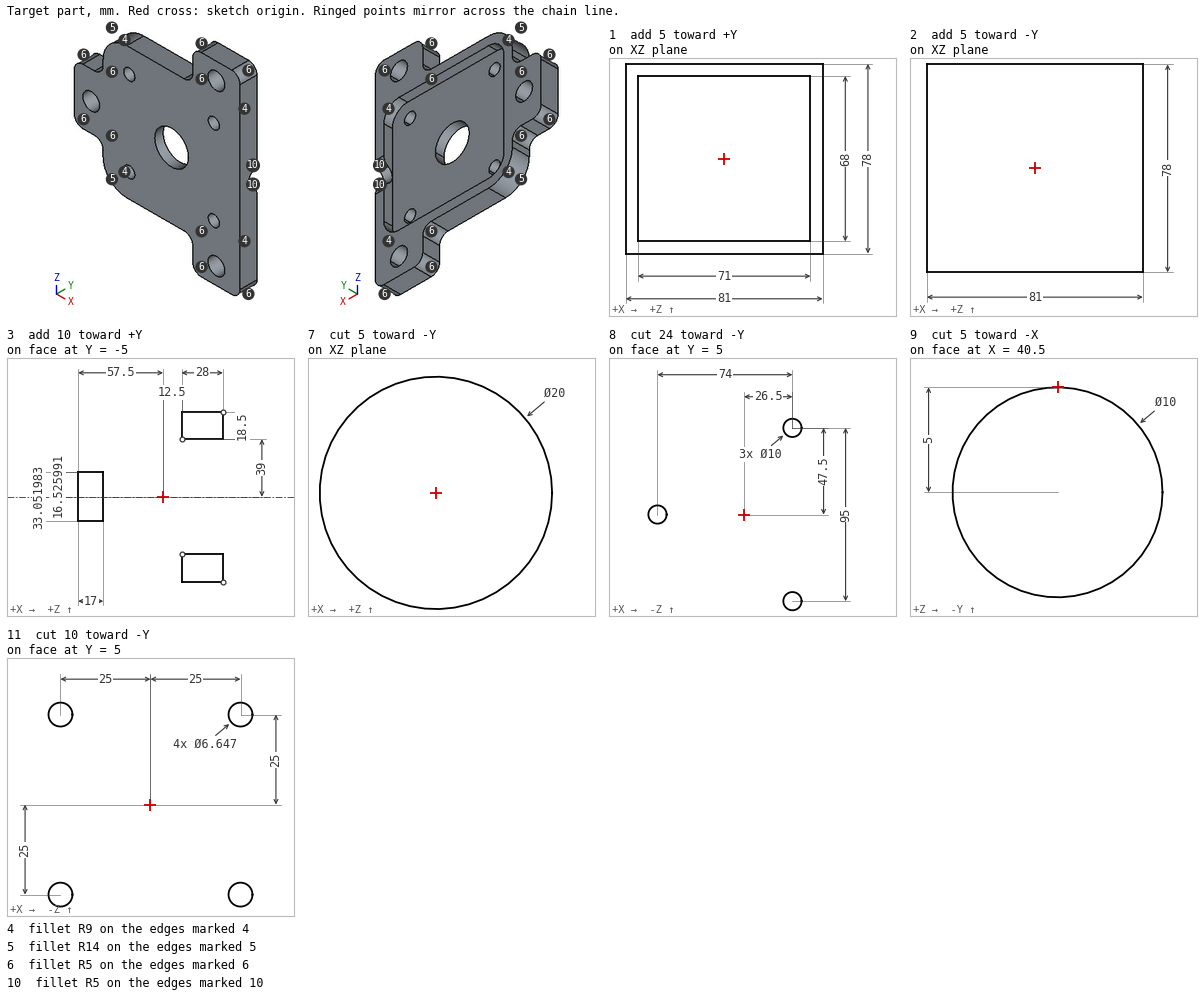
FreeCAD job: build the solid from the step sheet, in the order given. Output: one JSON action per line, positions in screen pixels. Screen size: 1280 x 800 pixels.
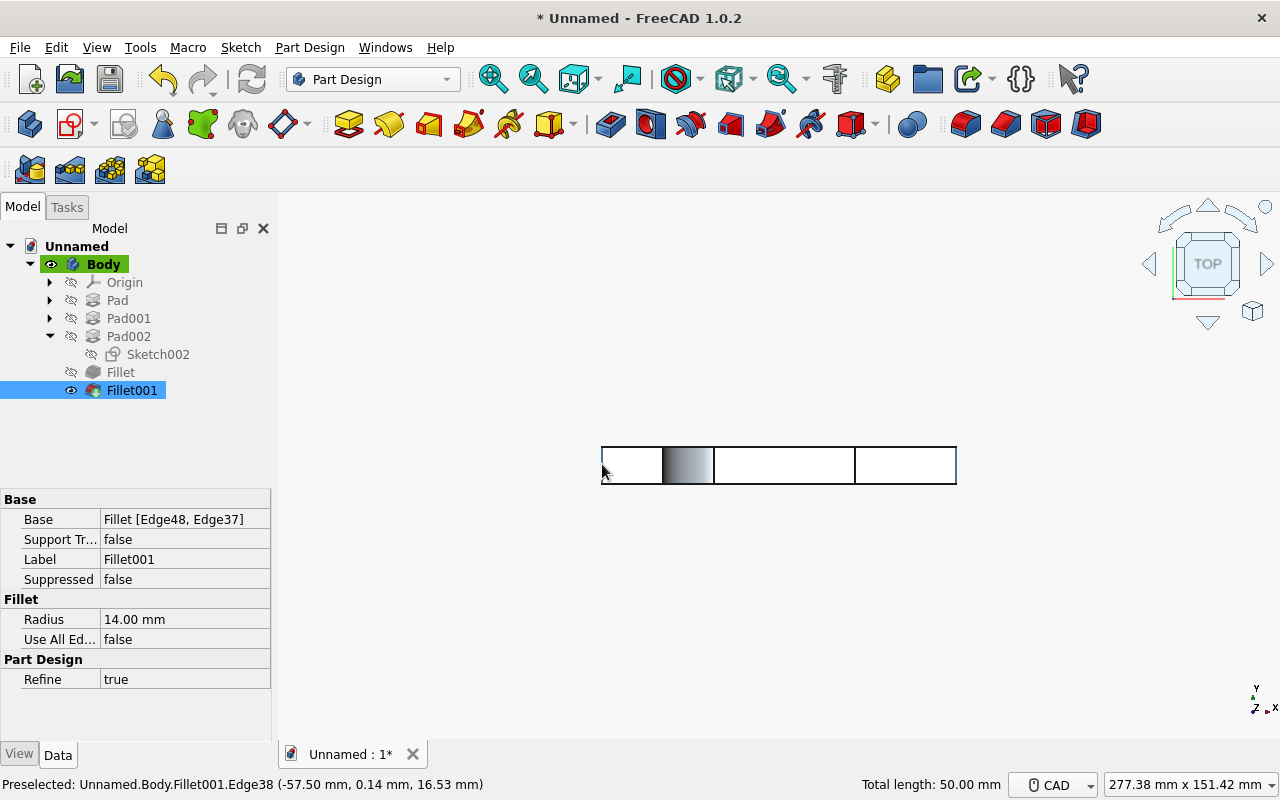
{"action": "left_click", "coordinate": [855, 464], "text": "ctrl"}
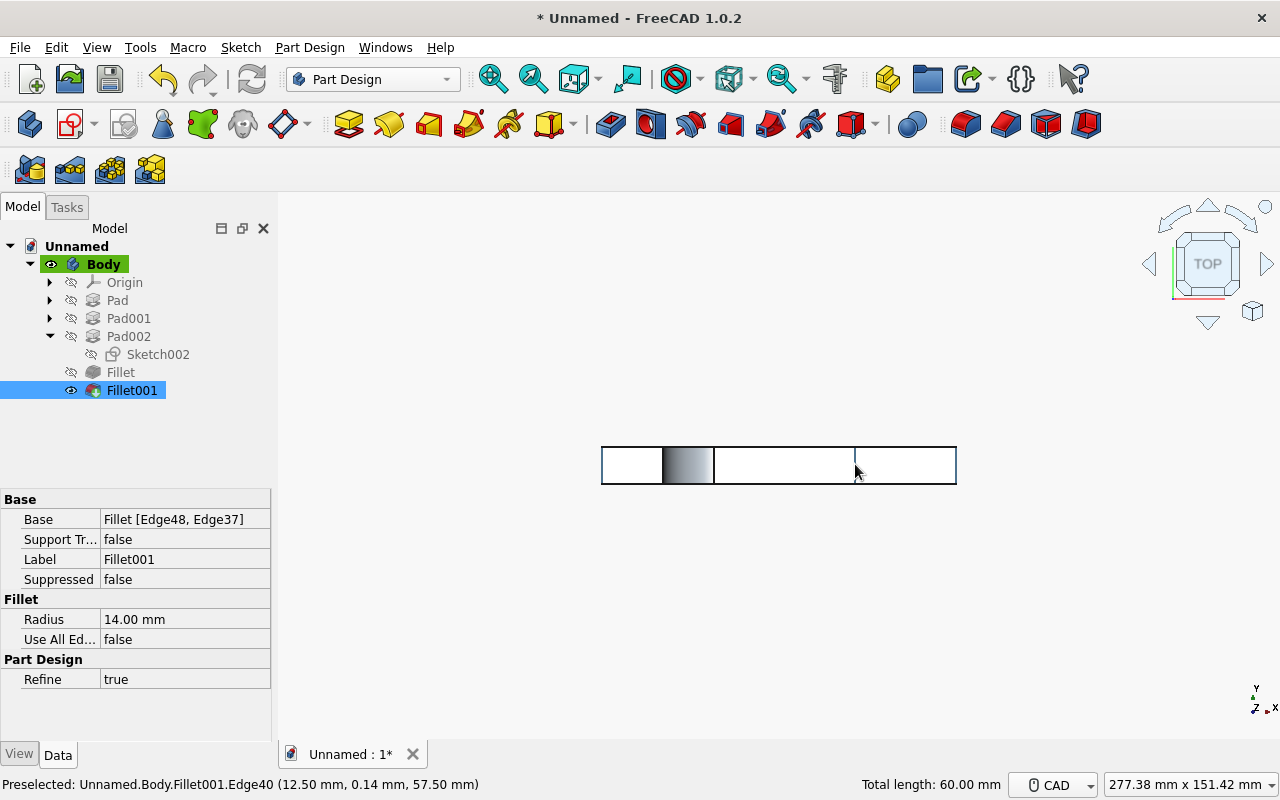
{"action": "key", "text": "1"}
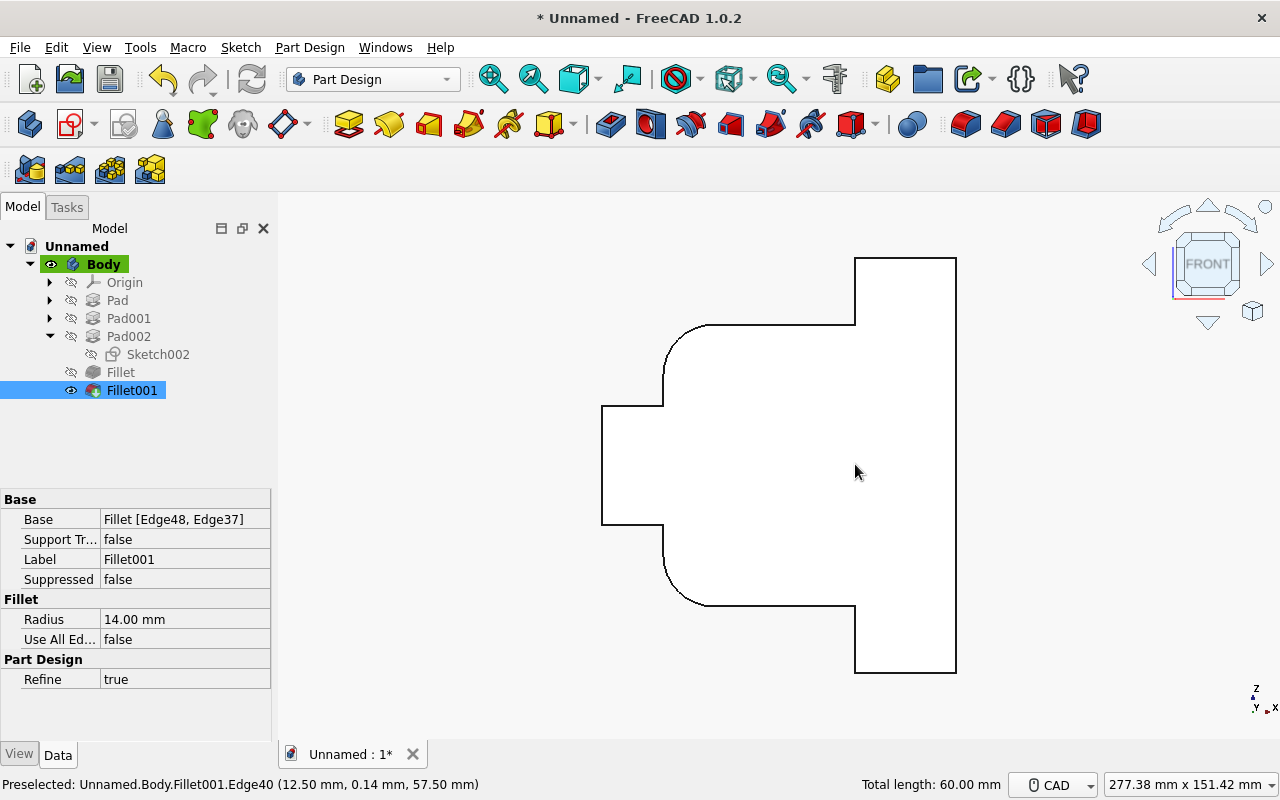
{"action": "key", "text": "3"}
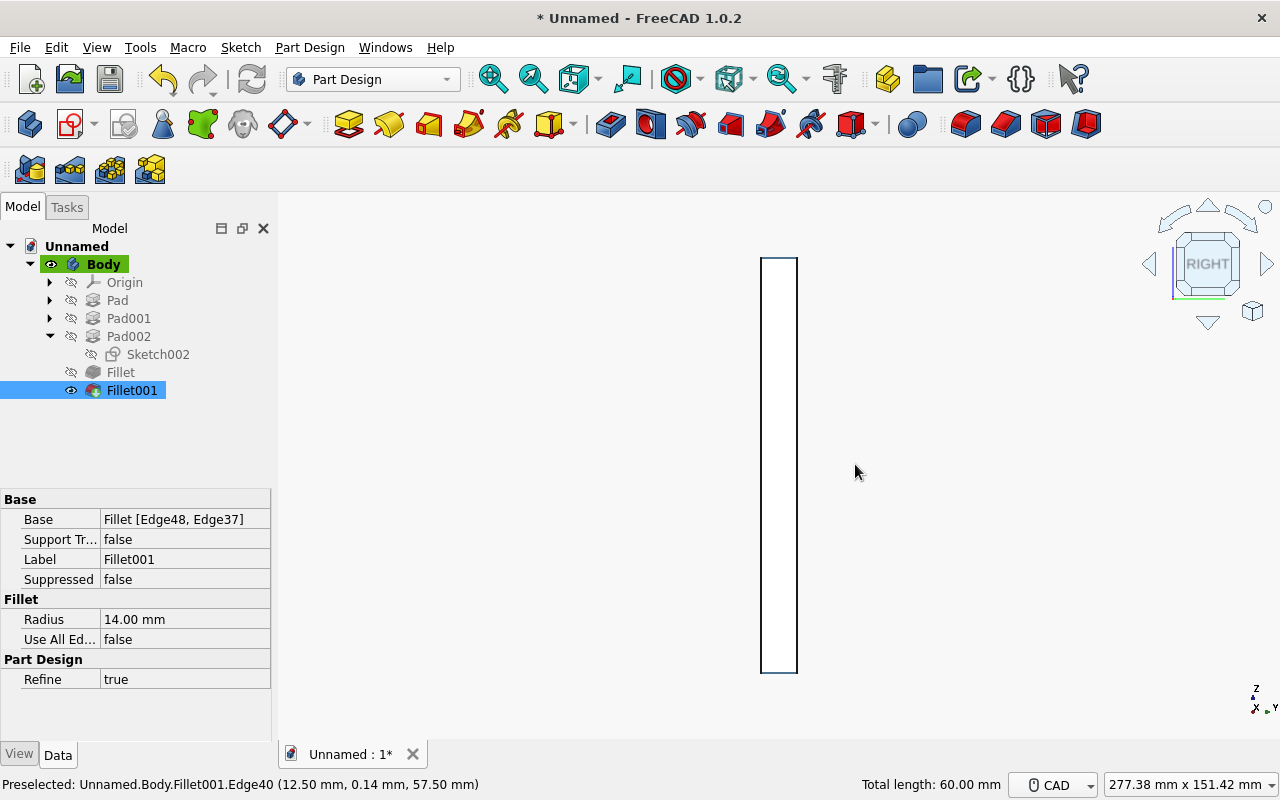
{"action": "key", "text": "5"}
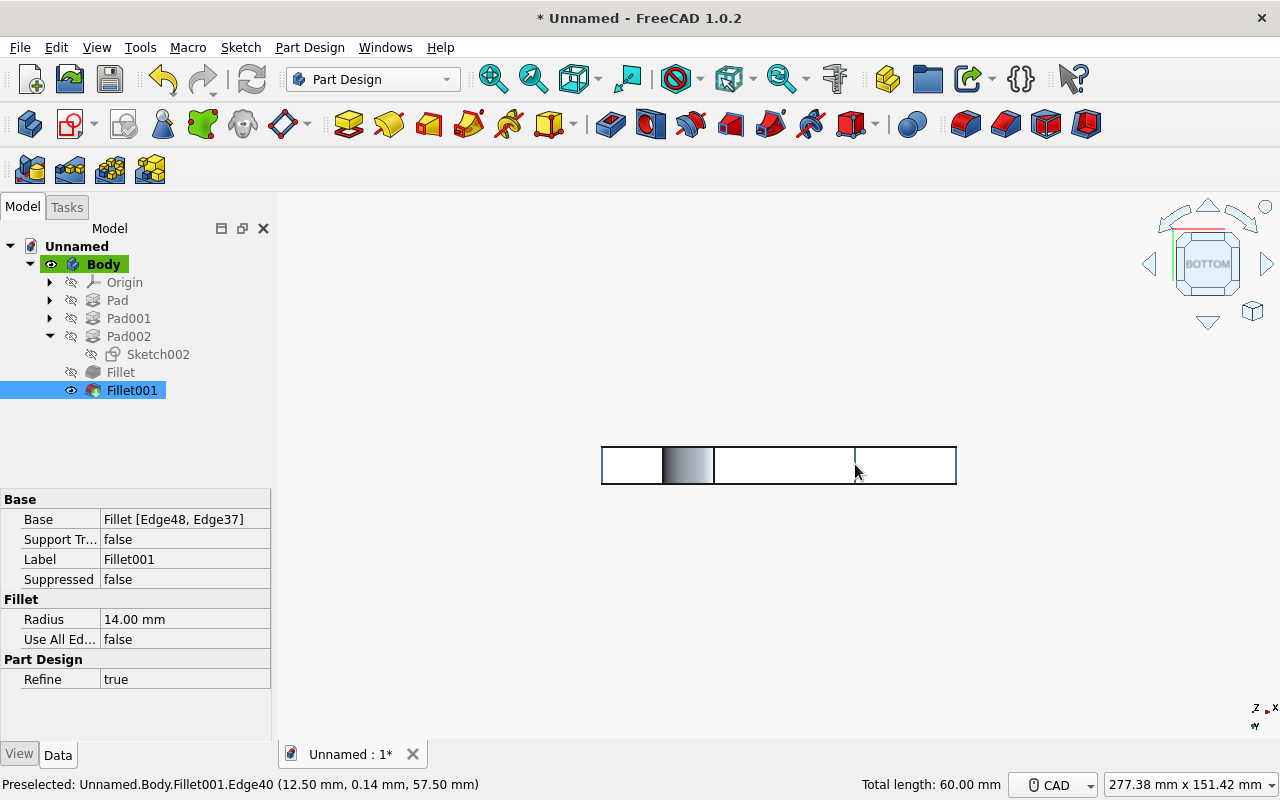
{"action": "key", "text": "v f"}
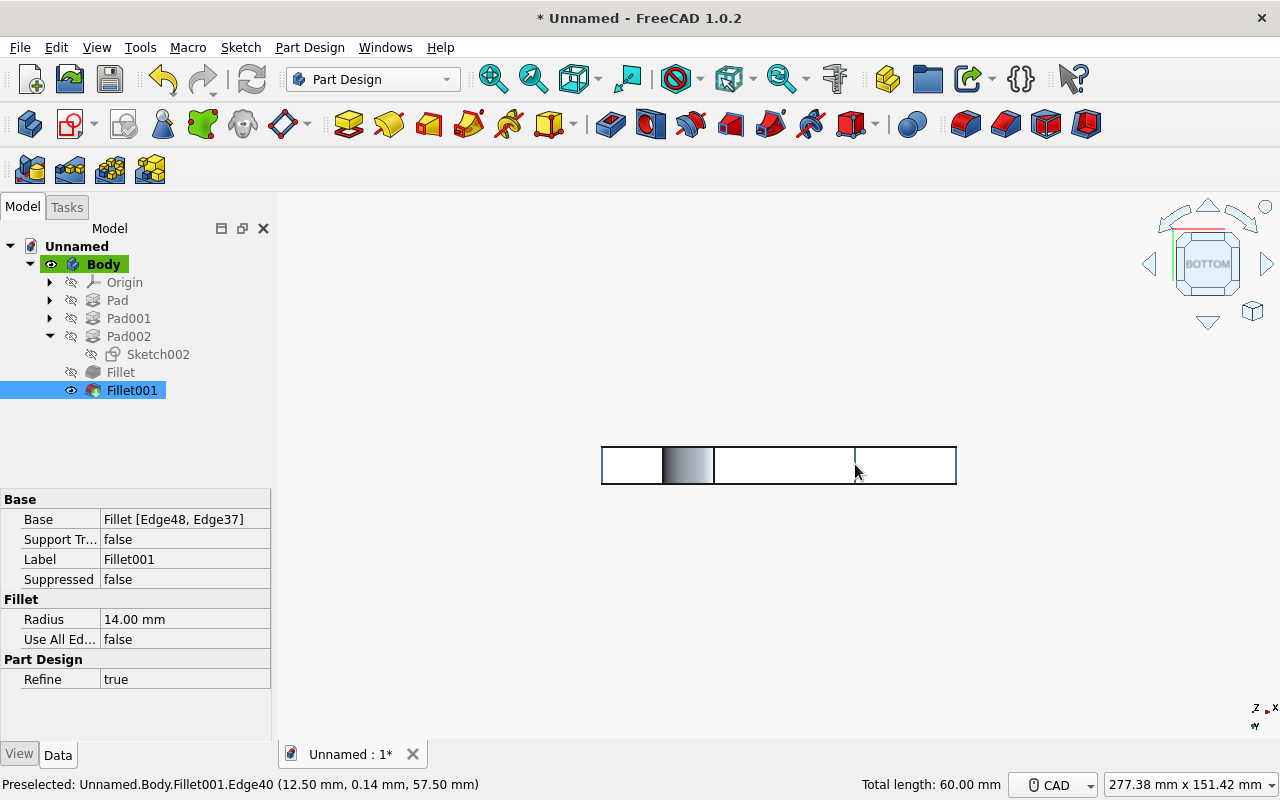
{"action": "key", "text": "4"}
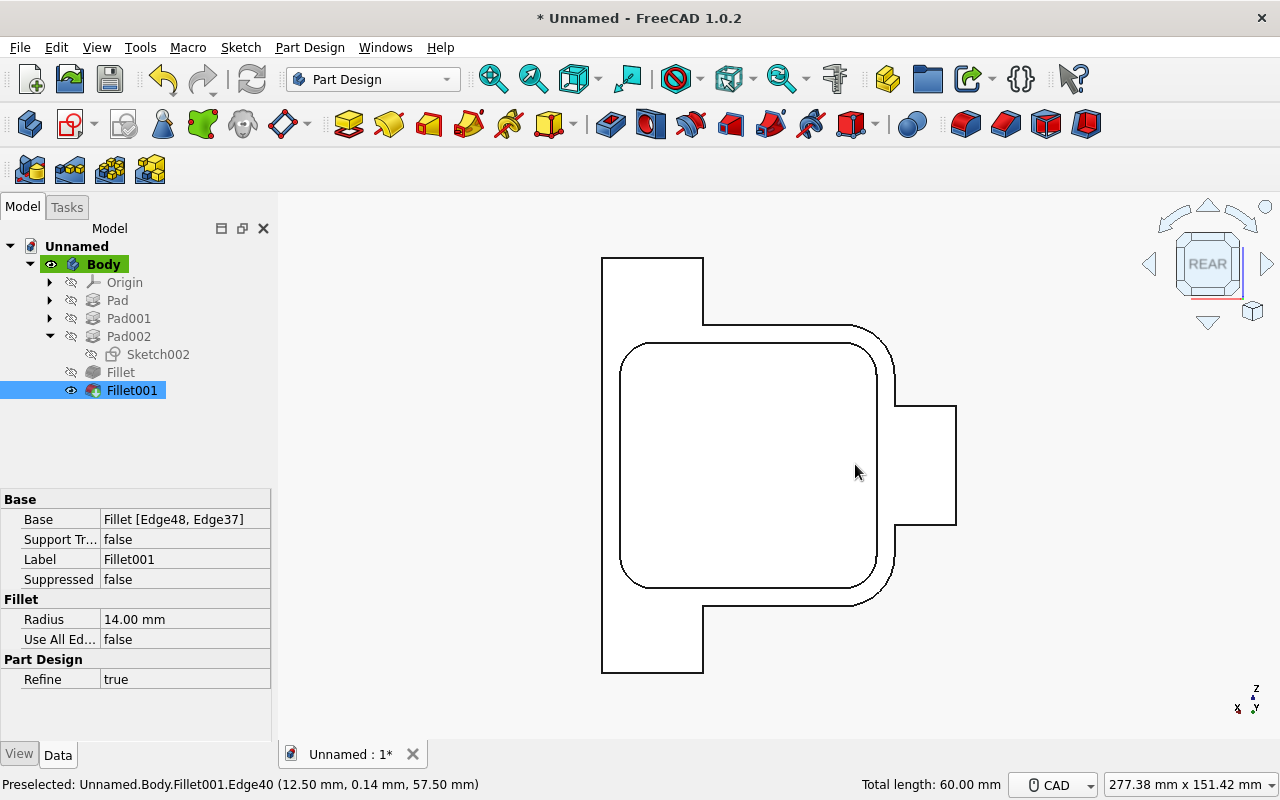
{"action": "key", "text": "6"}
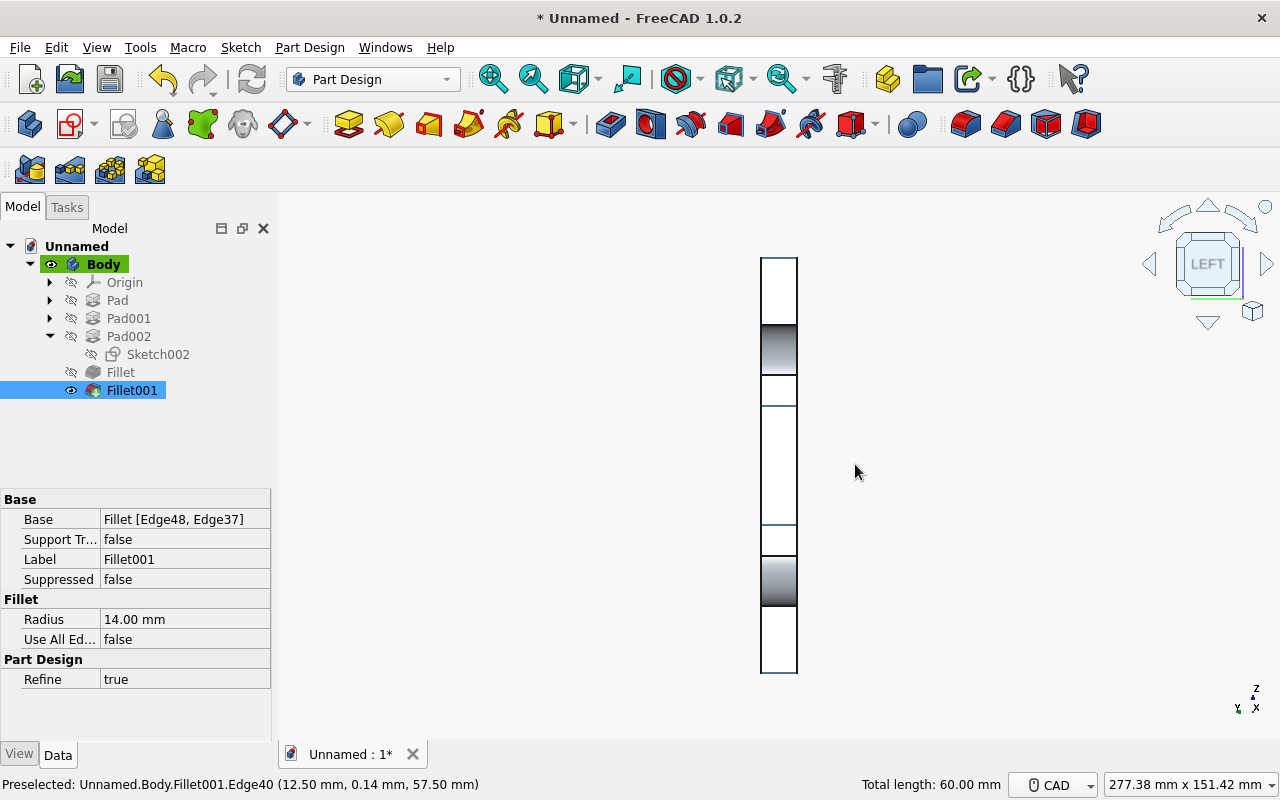
{"action": "key", "text": "v 3"}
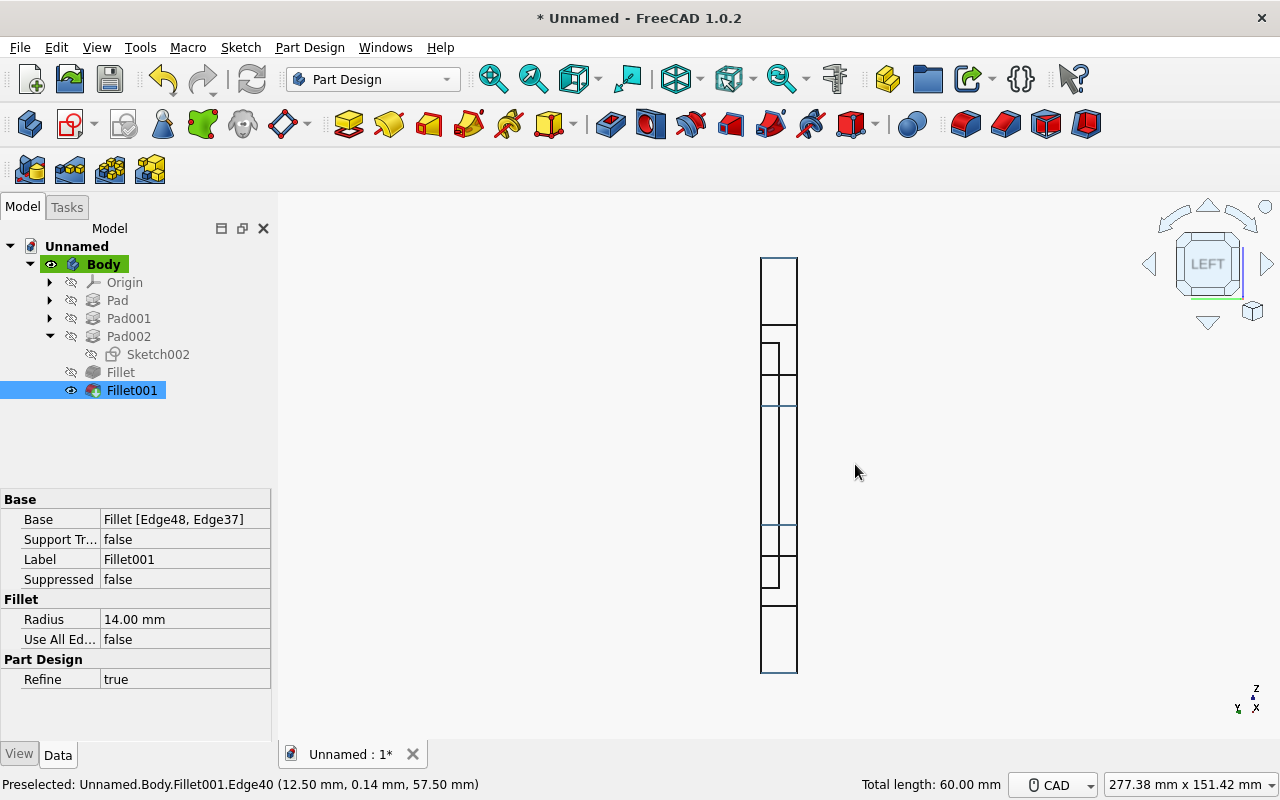
{"action": "key", "text": "0"}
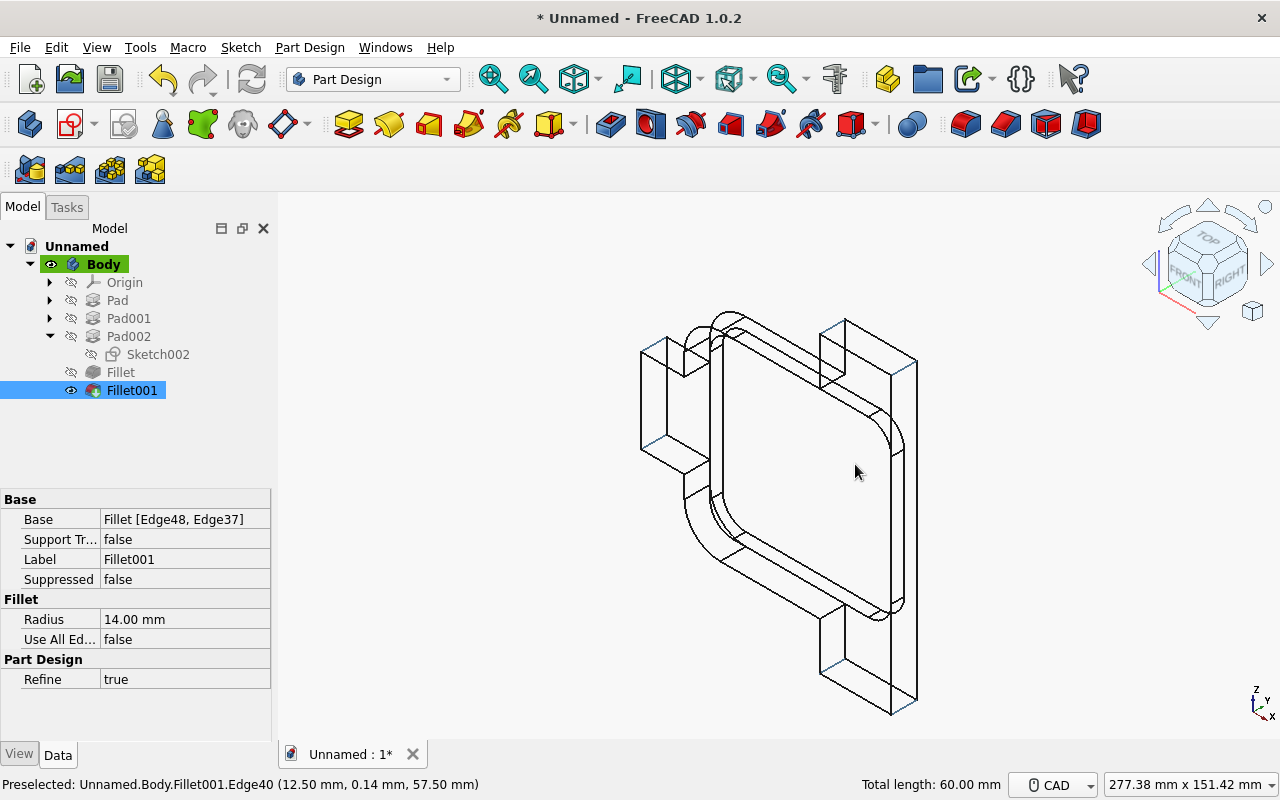
{"action": "left_click", "coordinate": [697, 369], "text": "ctrl"}